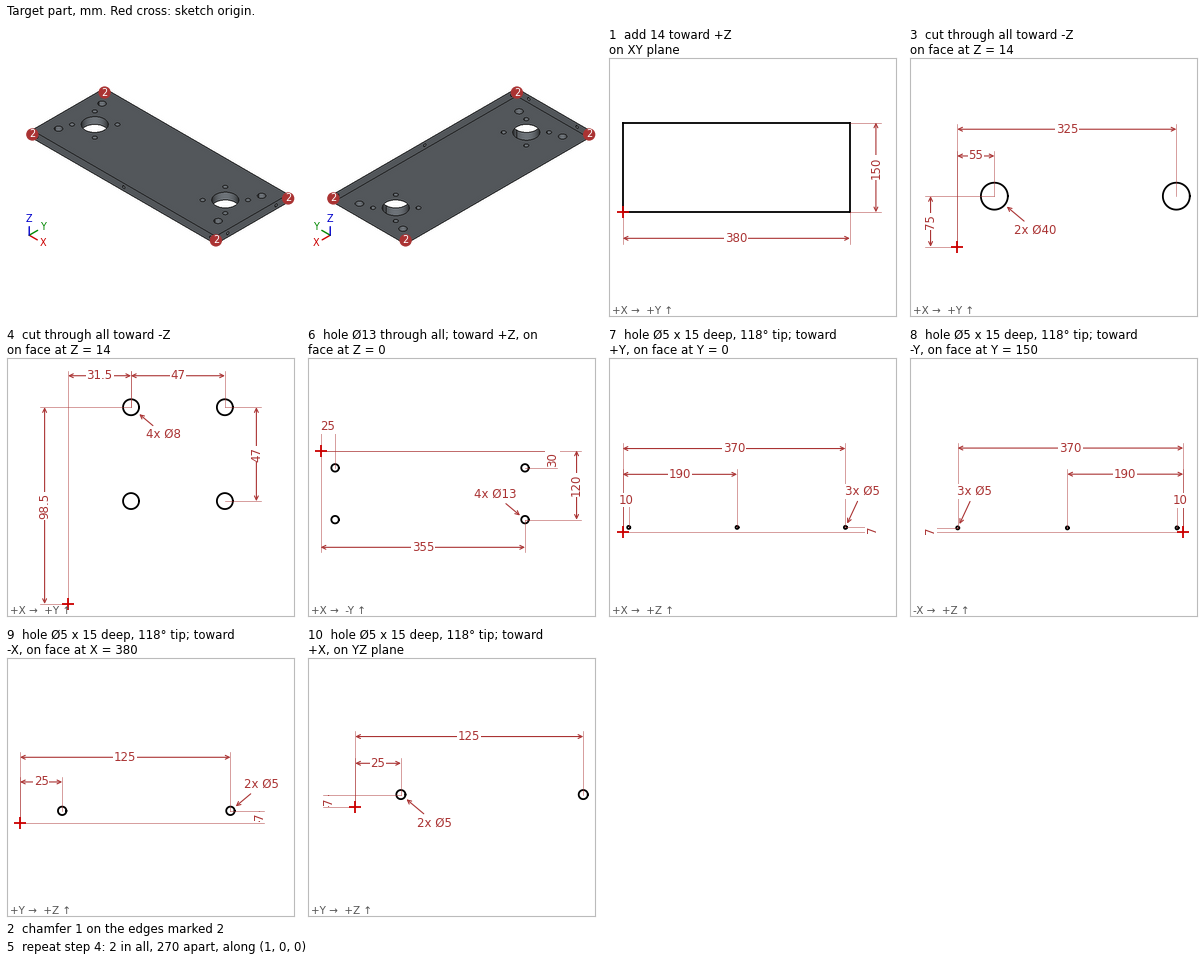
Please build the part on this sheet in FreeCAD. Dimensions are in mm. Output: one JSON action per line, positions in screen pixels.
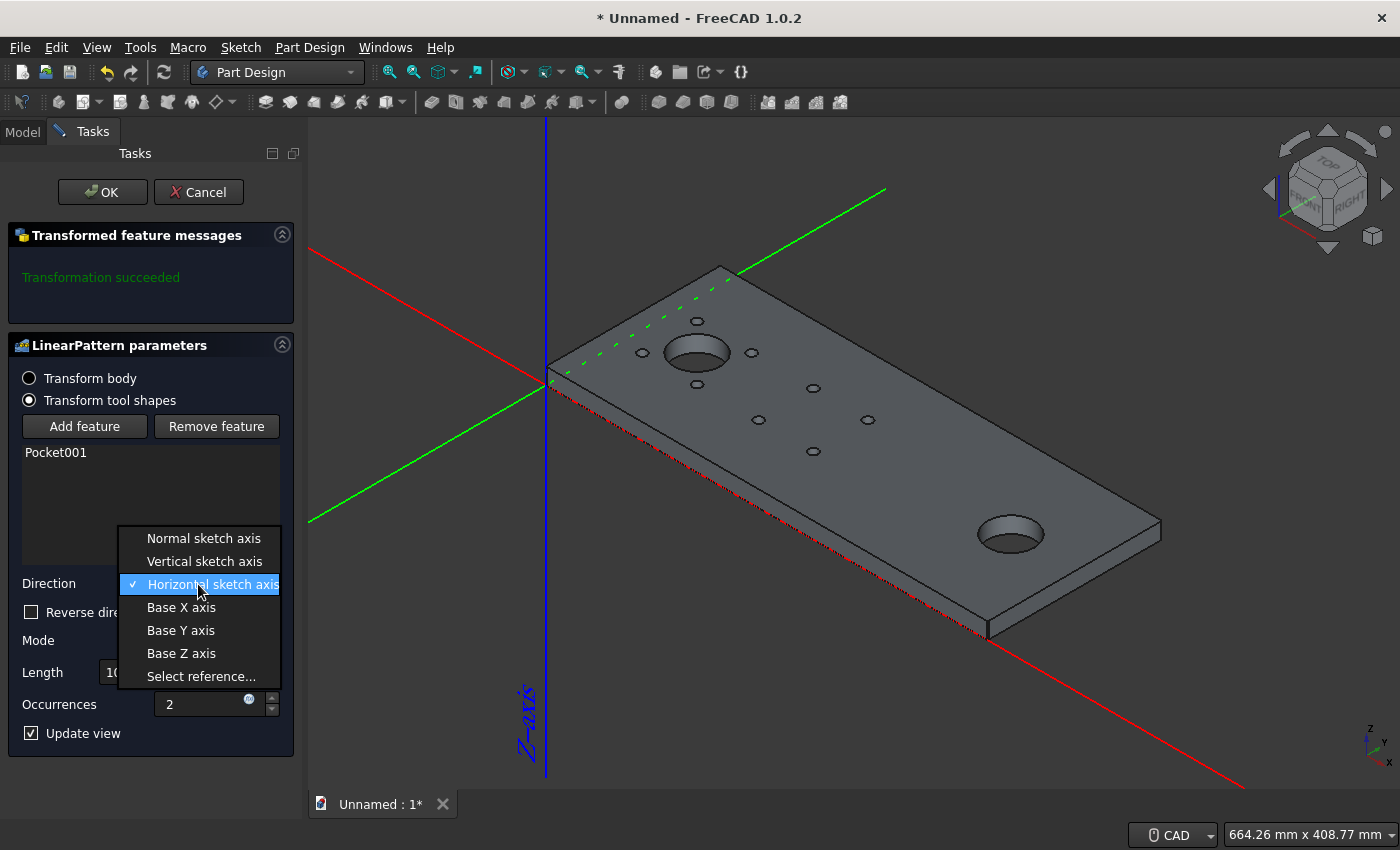
{"action": "left_click", "coordinate": [198, 608]}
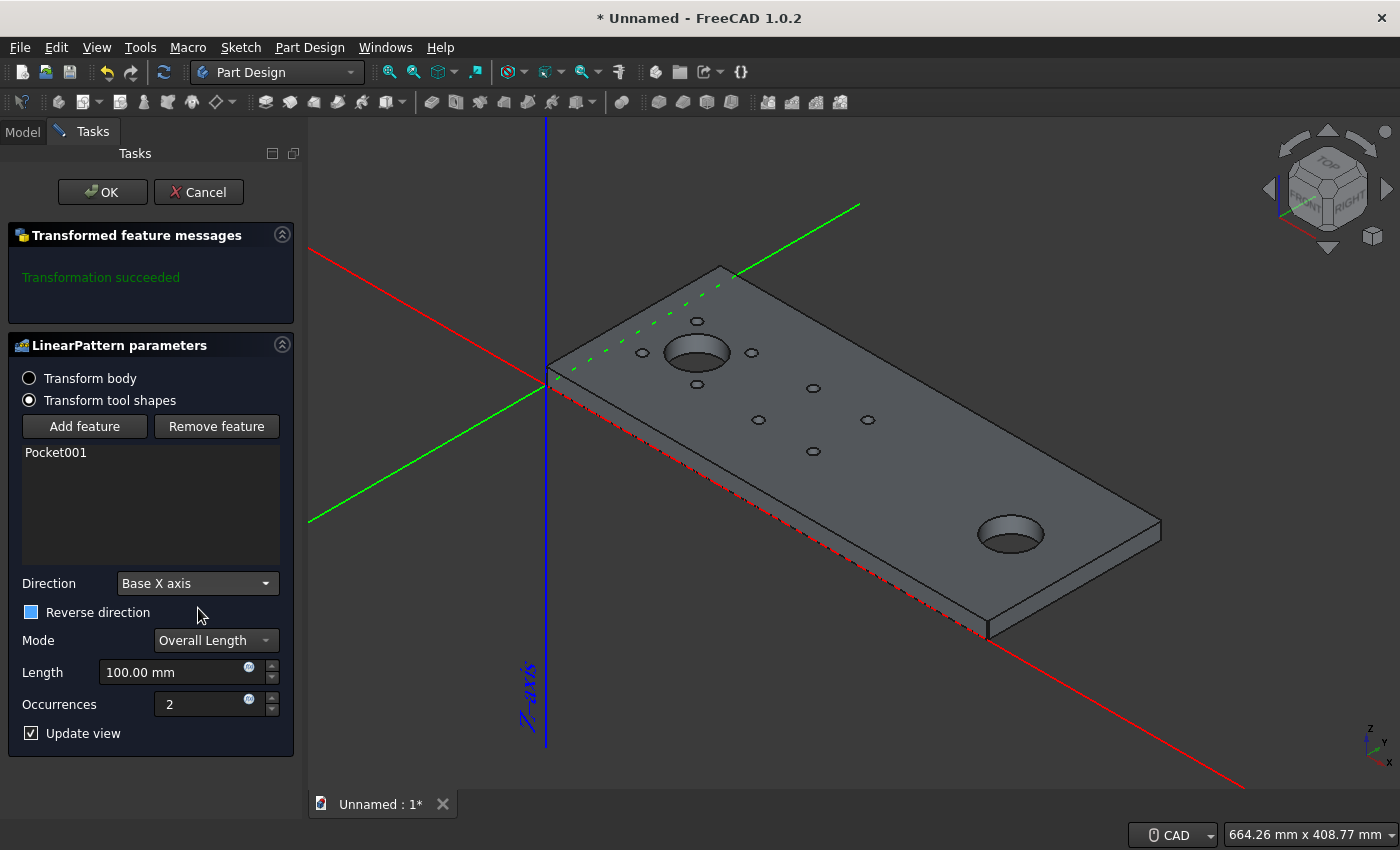
{"action": "left_click", "coordinate": [217, 640]}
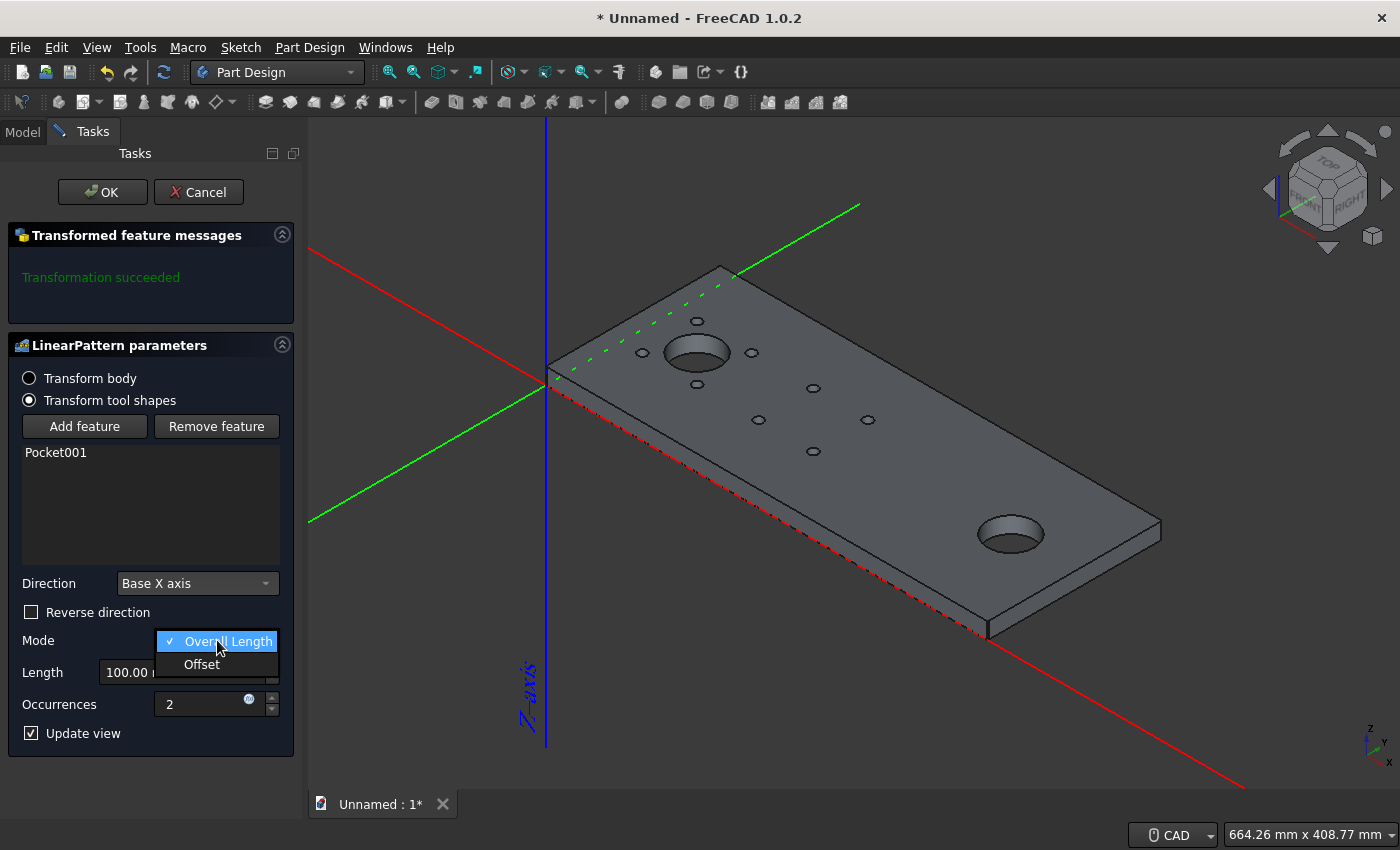
{"action": "left_click", "coordinate": [216, 664]}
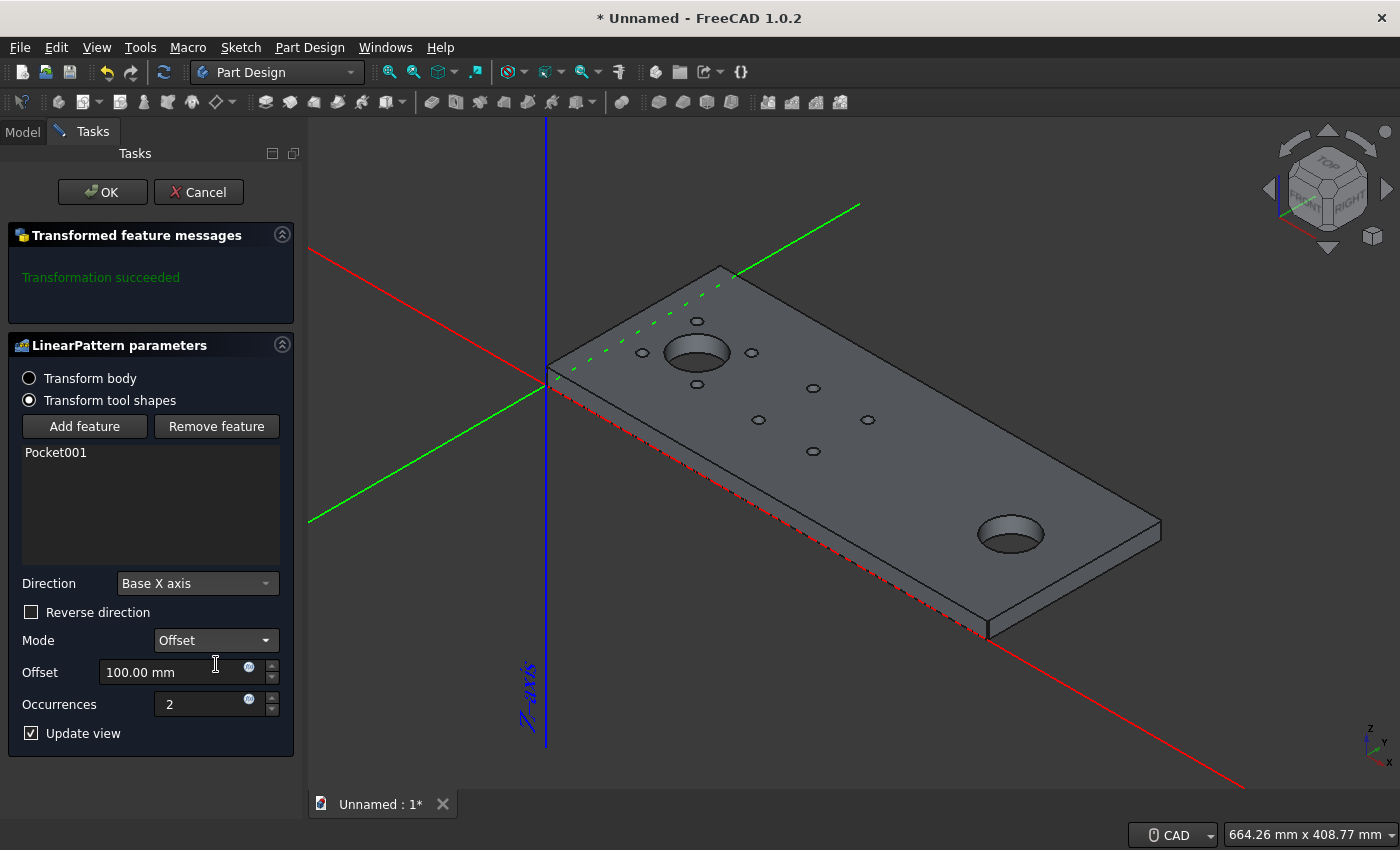
{"action": "triple_click", "coordinate": [182, 672]}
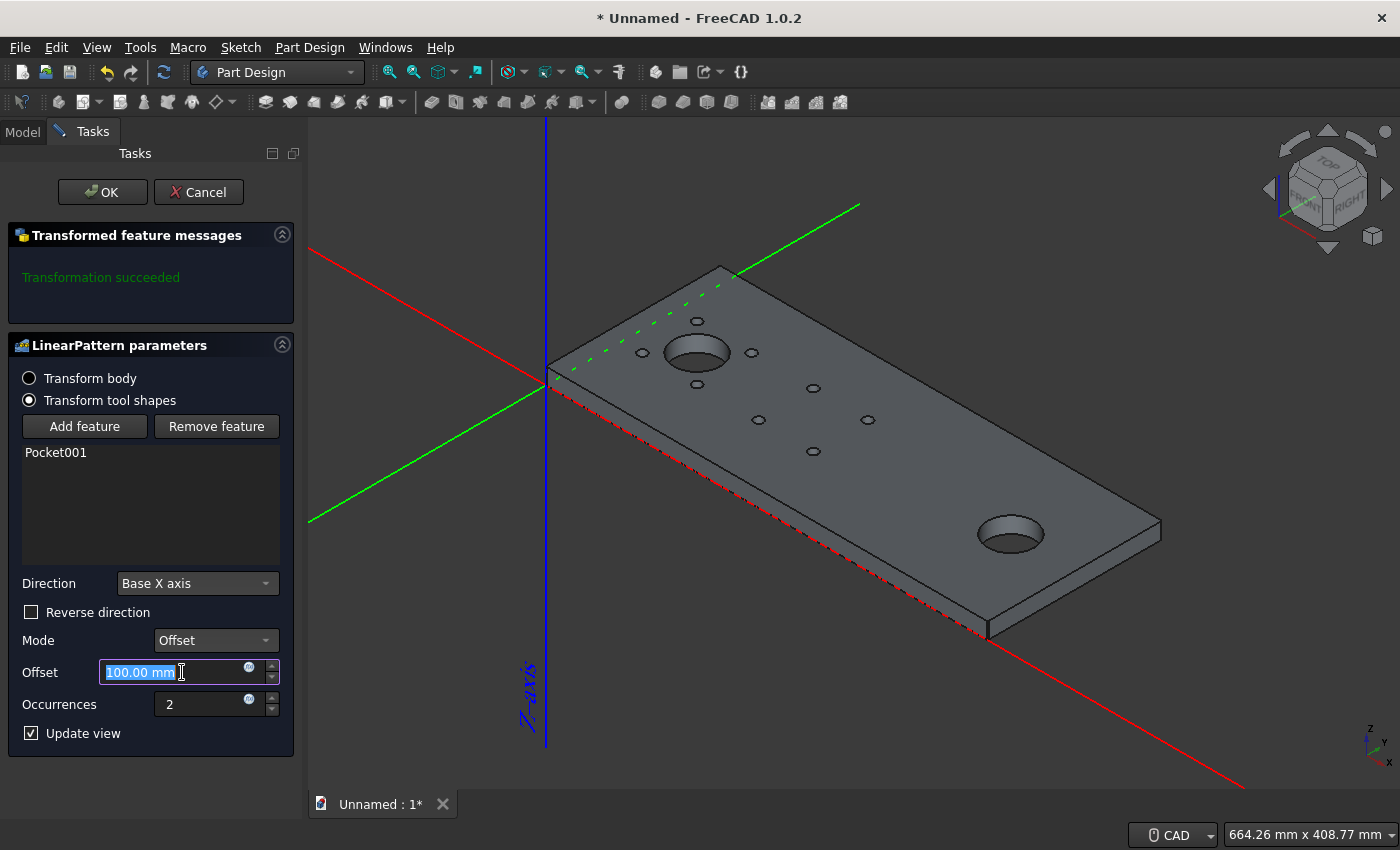
{"action": "type", "text": "270"}
{"action": "key", "text": "Tab"}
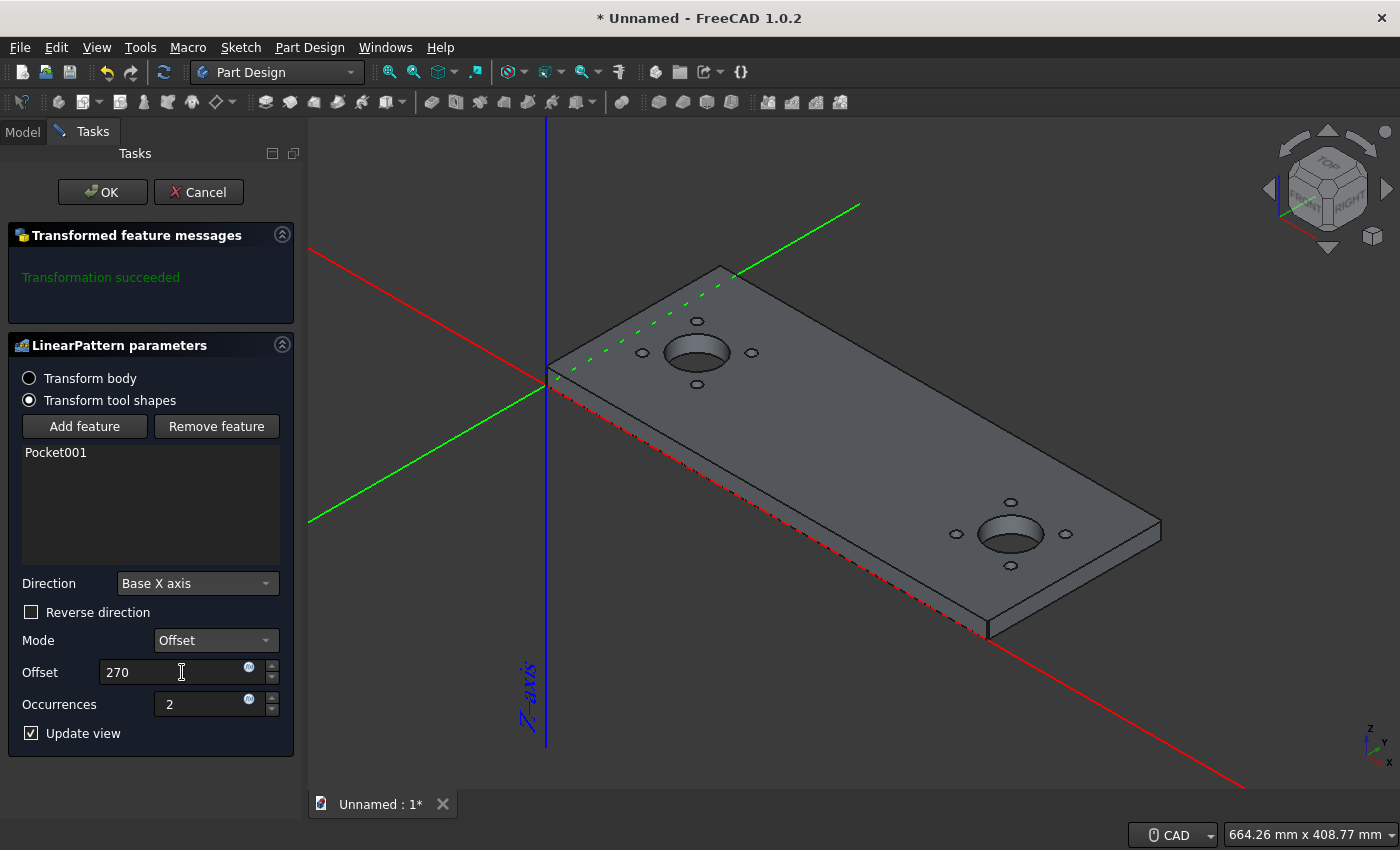
{"action": "triple_click", "coordinate": [209, 704]}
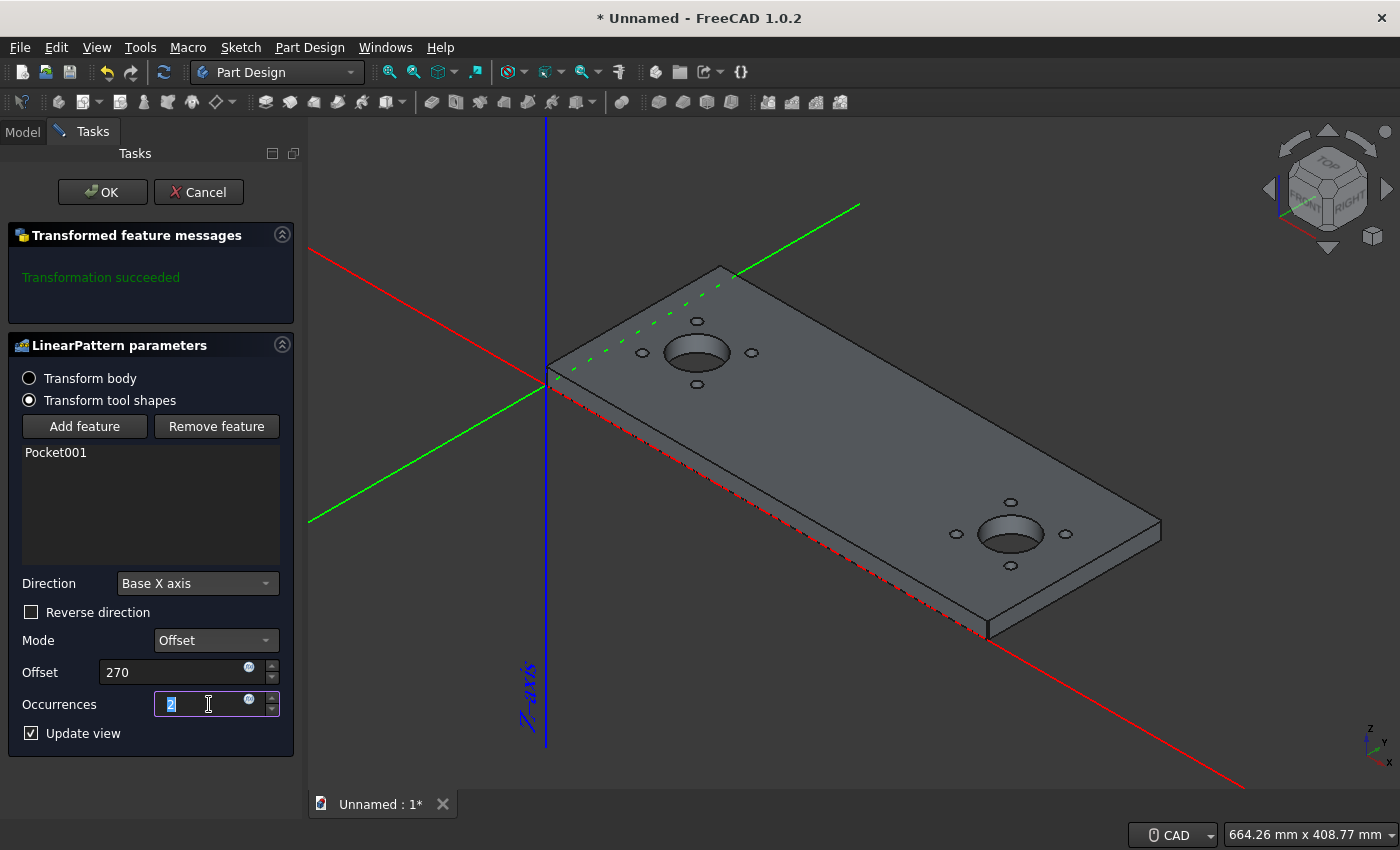
{"action": "type", "text": "2"}
{"action": "key", "text": "Tab"}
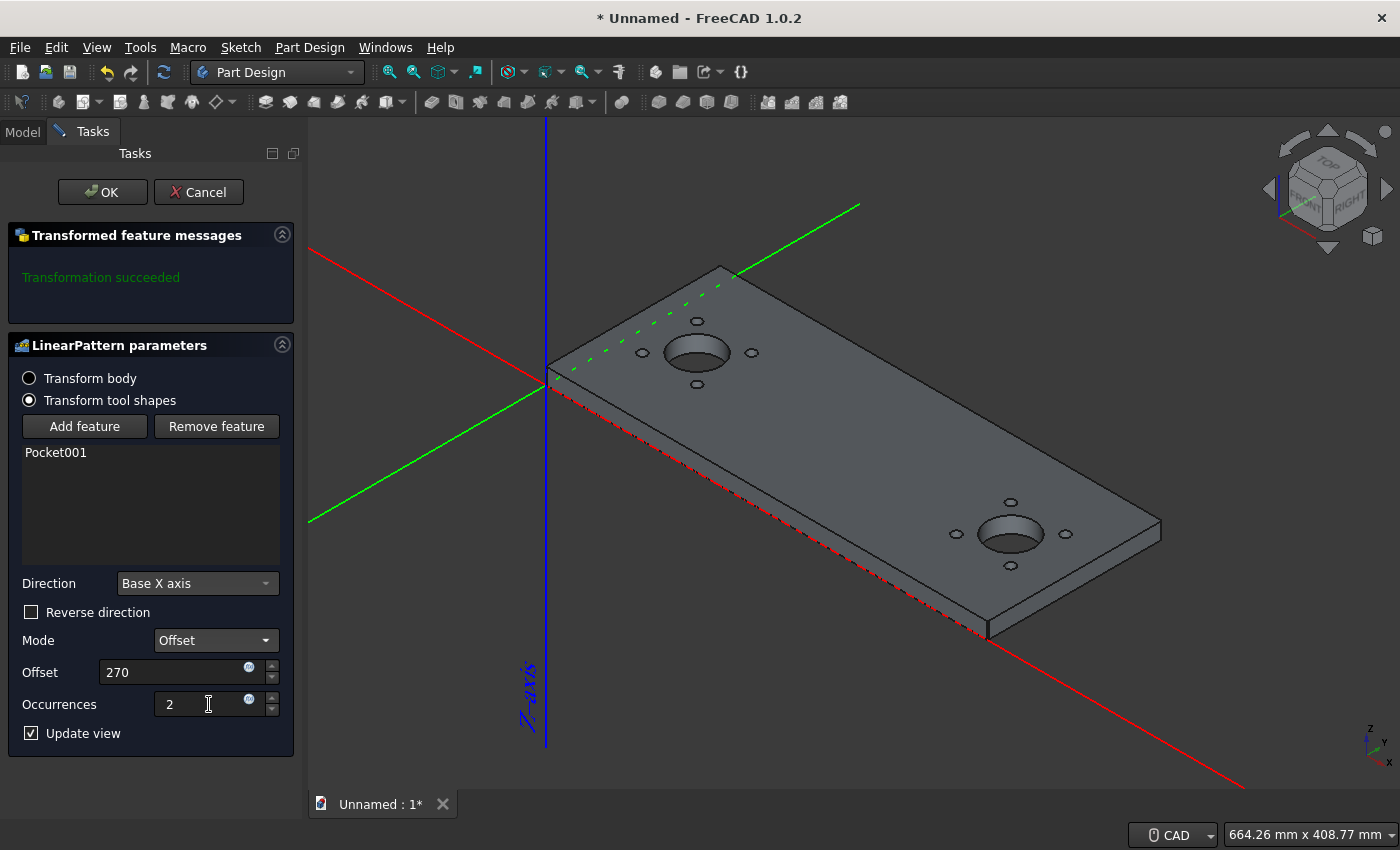
{"action": "left_click", "coordinate": [103, 192]}